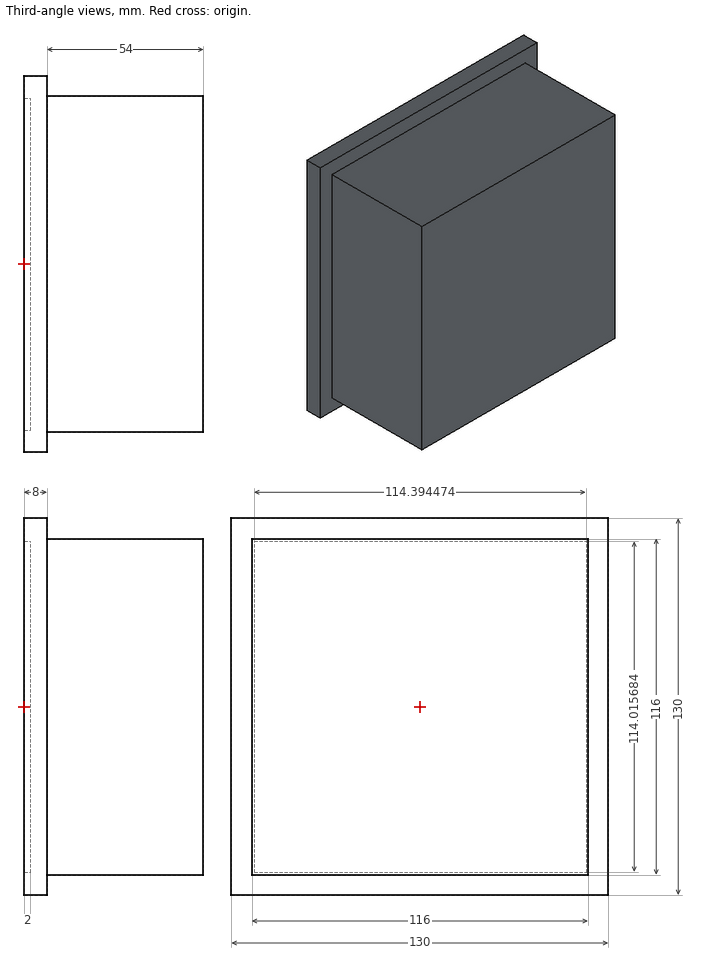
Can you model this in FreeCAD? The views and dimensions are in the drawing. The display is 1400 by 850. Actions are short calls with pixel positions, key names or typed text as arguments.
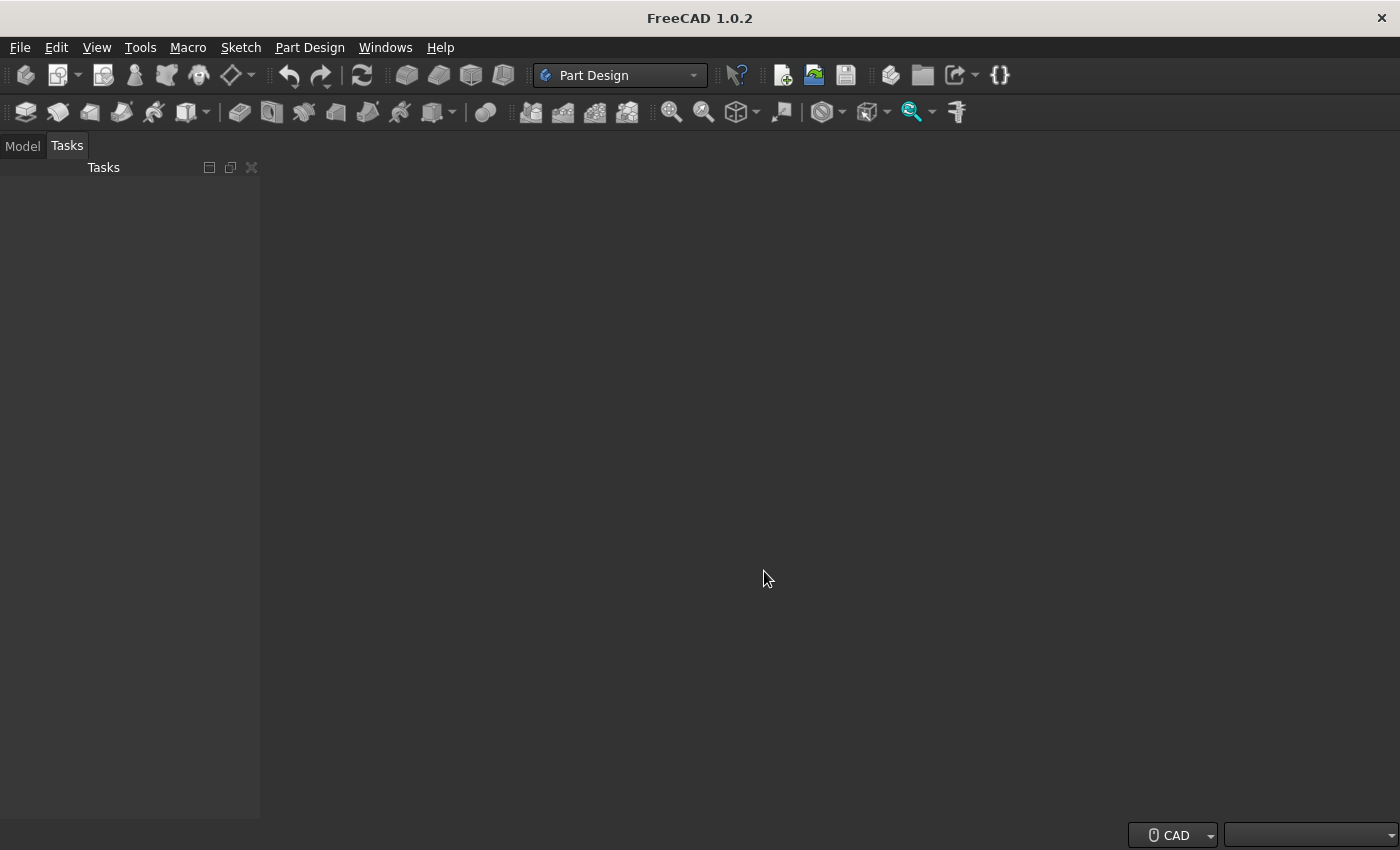
click(782, 76)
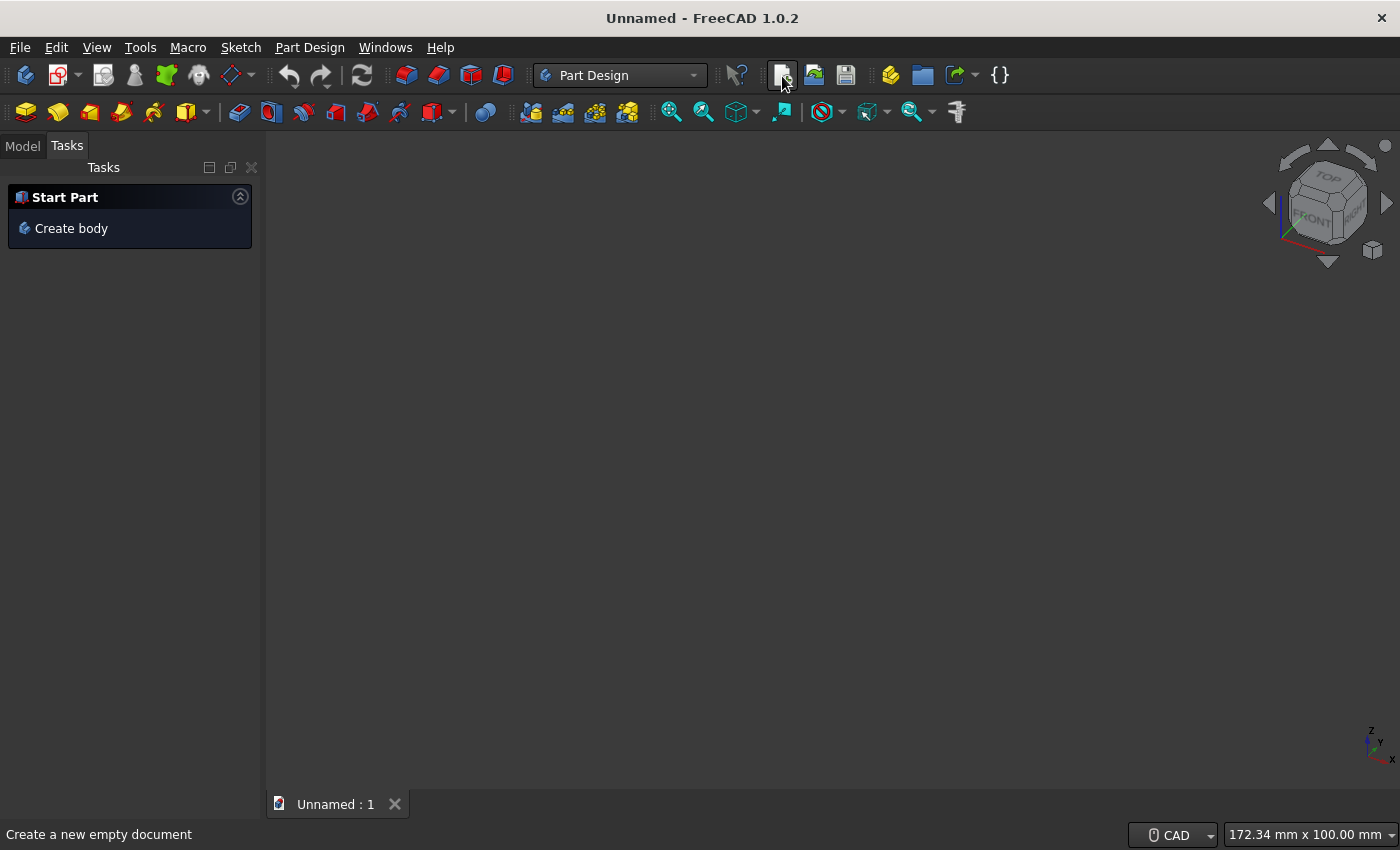
click(58, 76)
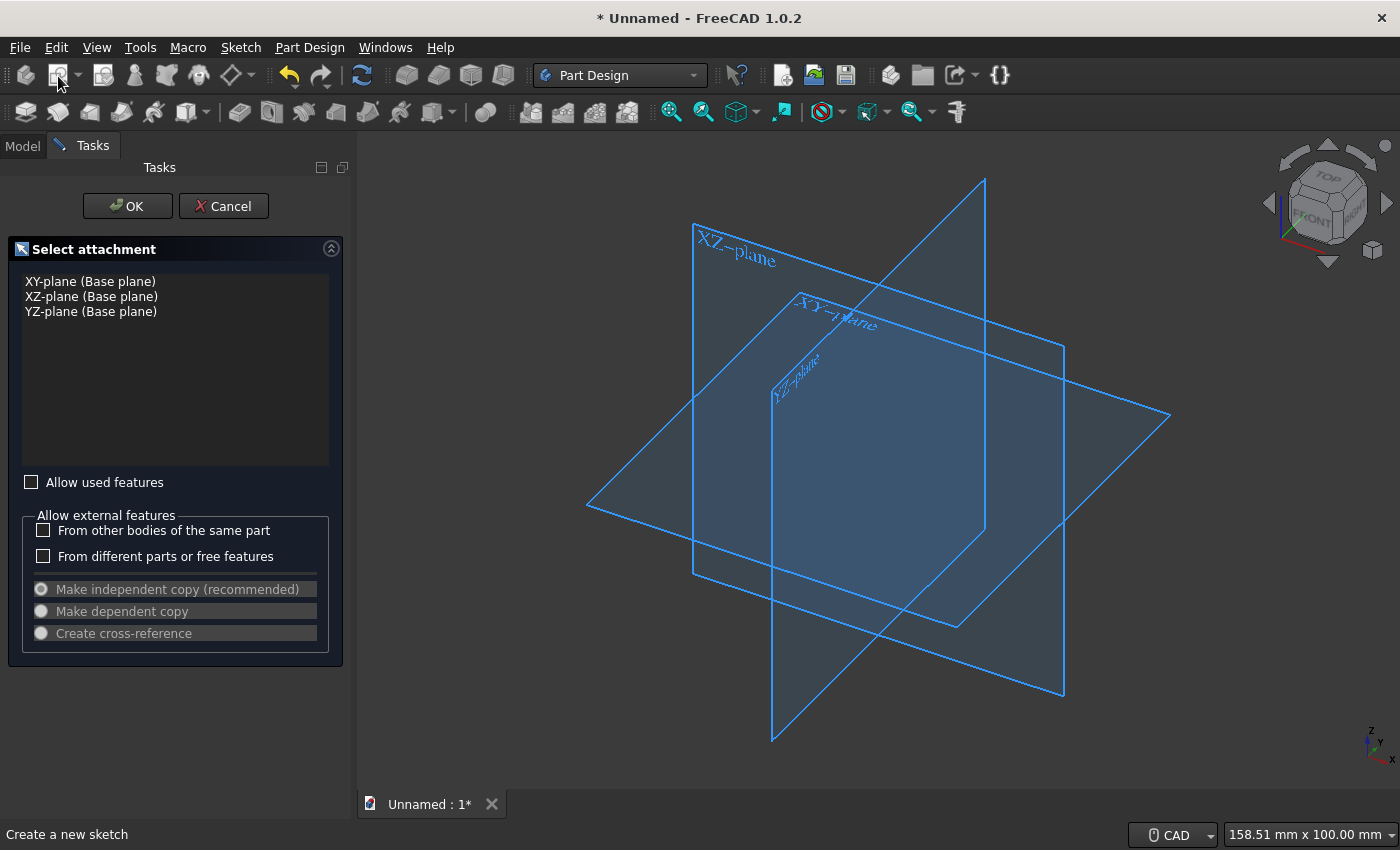
click(82, 312)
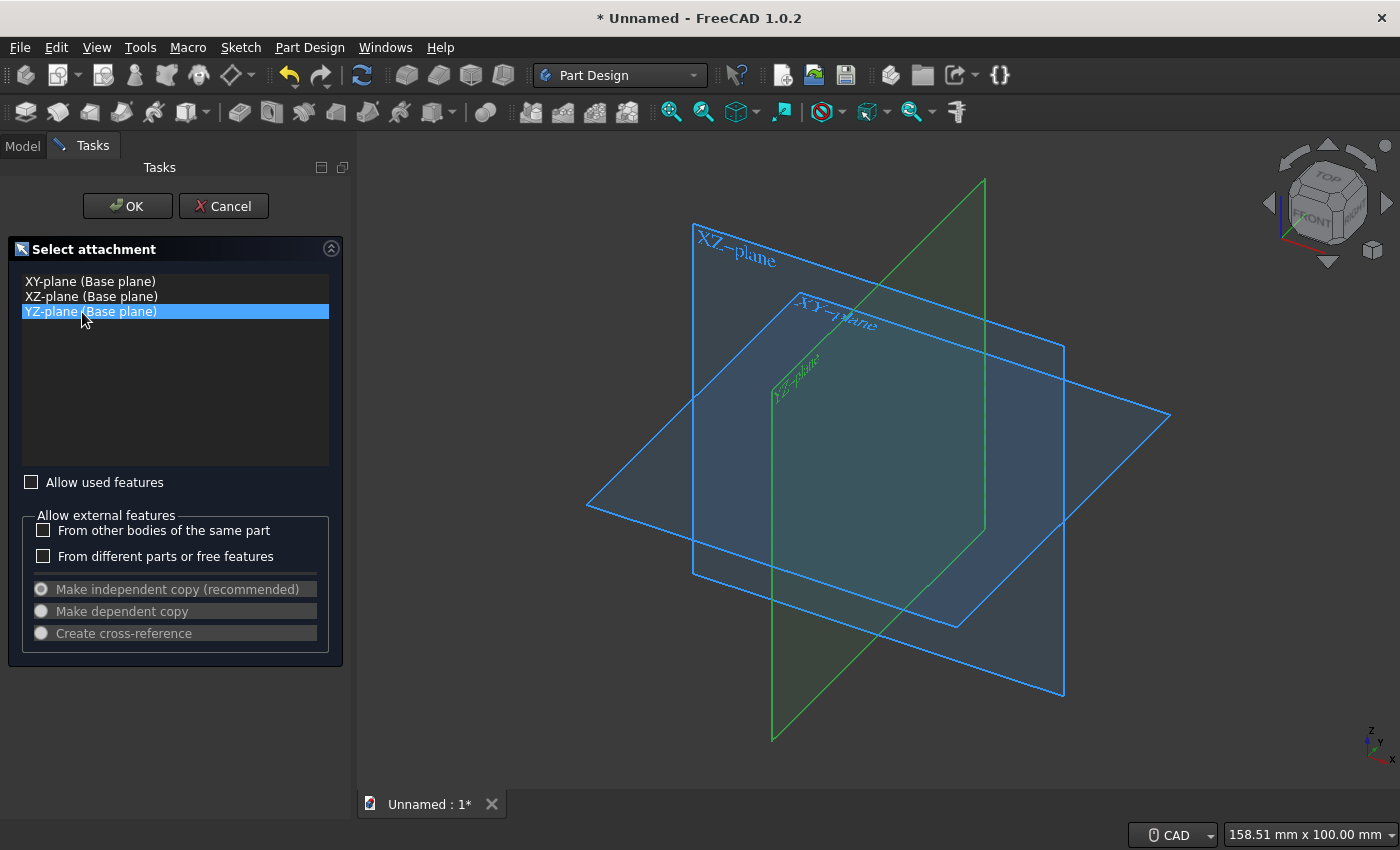
click(128, 206)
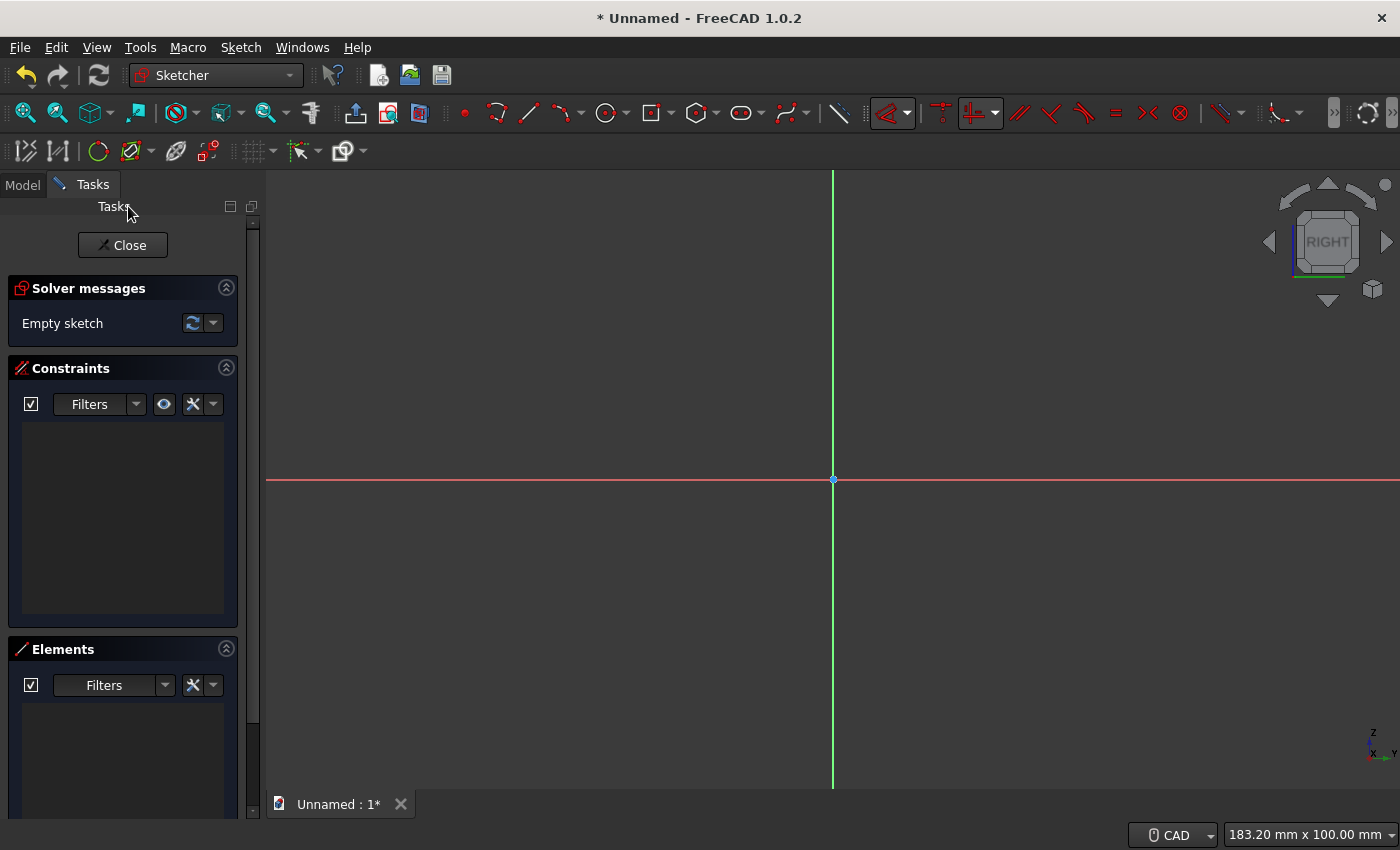
scroll(709, 480, down, 4)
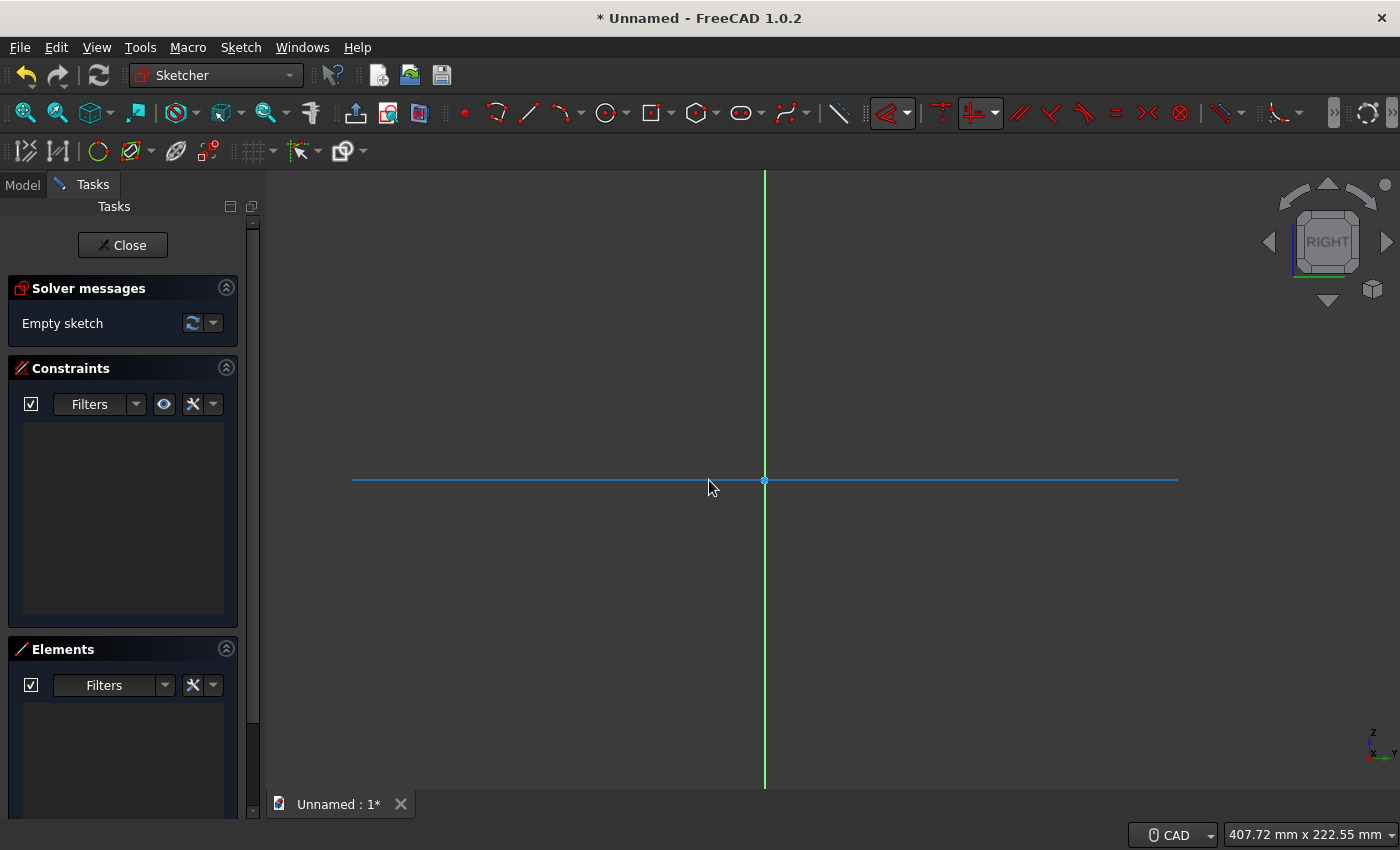
click(652, 114)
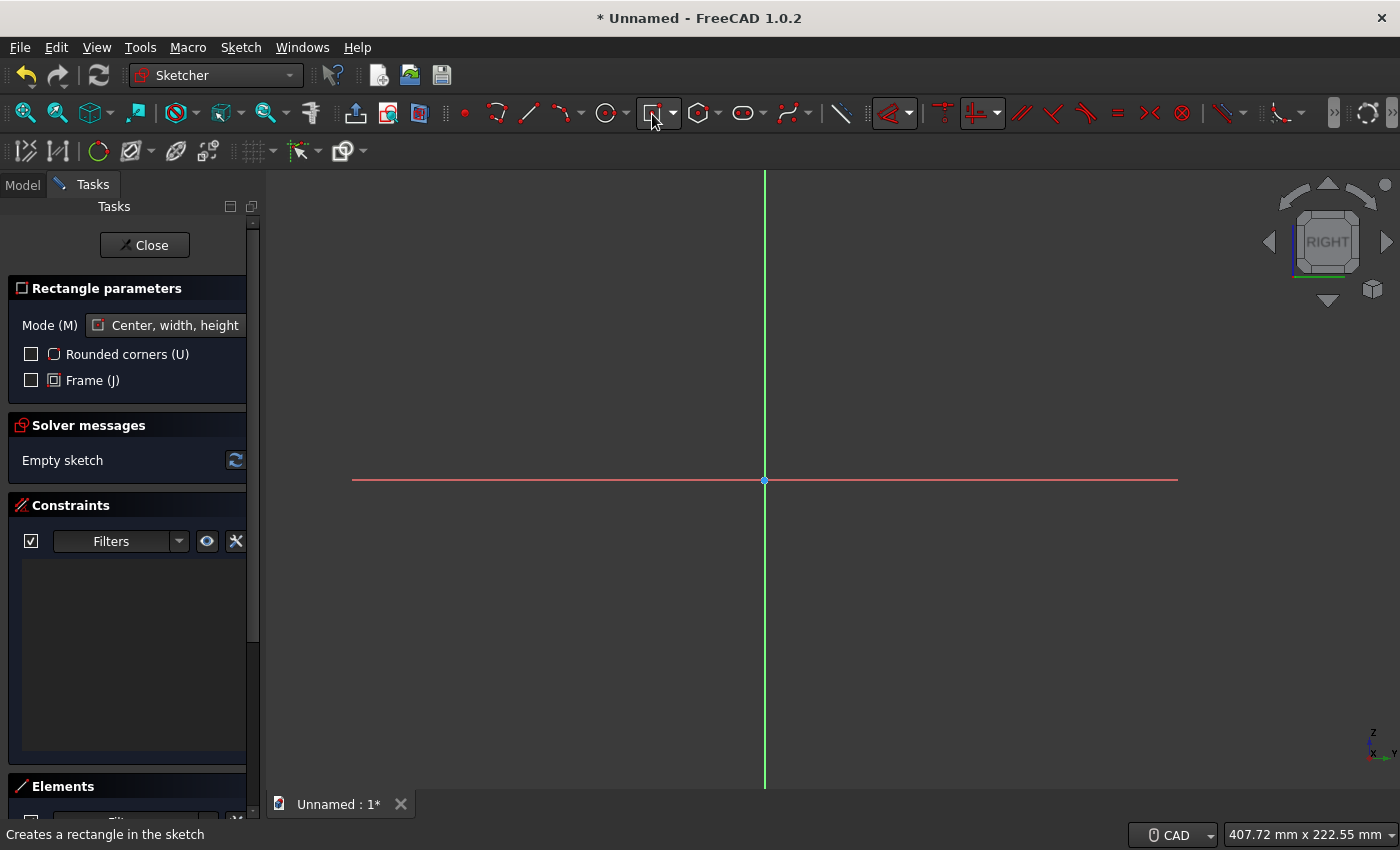
click(765, 480)
click(946, 299)
key(Escape)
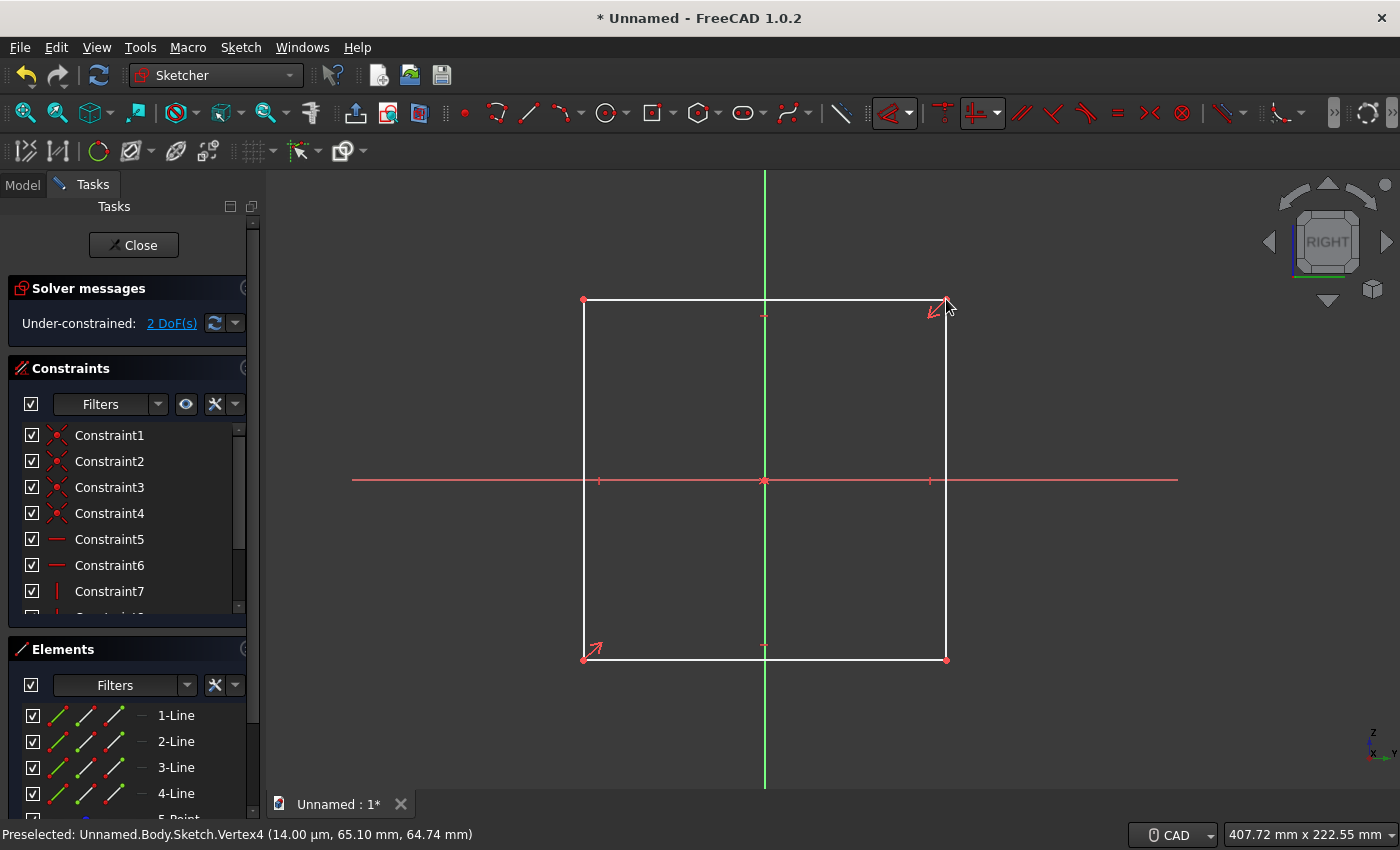
click(693, 660)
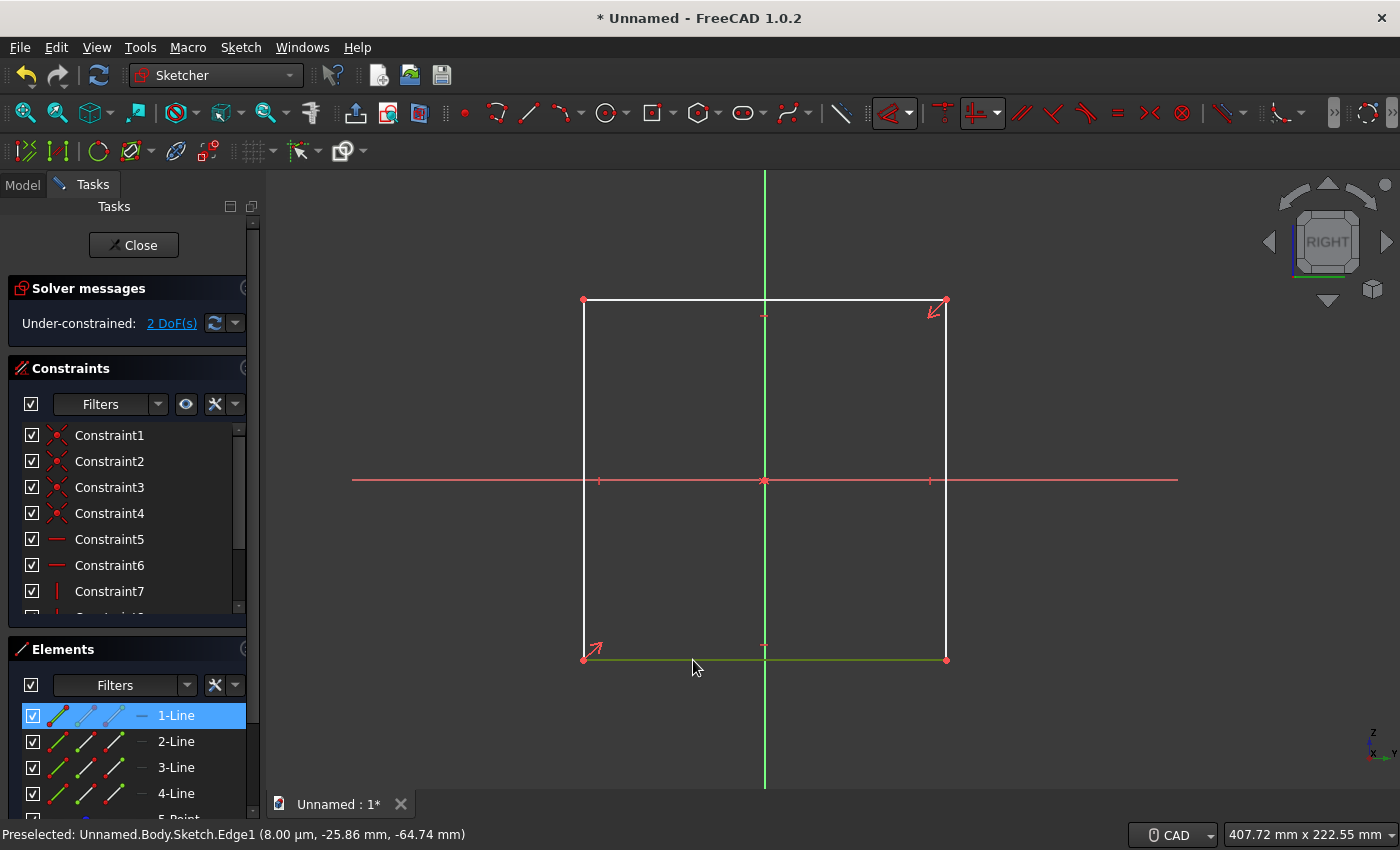
key(l)